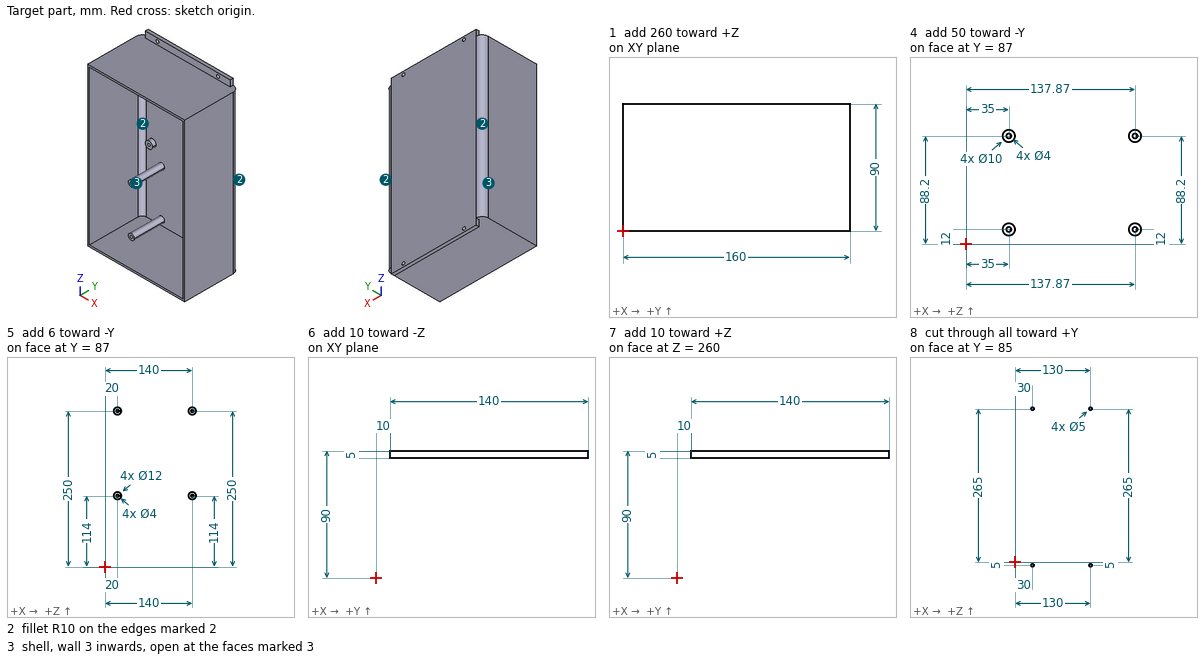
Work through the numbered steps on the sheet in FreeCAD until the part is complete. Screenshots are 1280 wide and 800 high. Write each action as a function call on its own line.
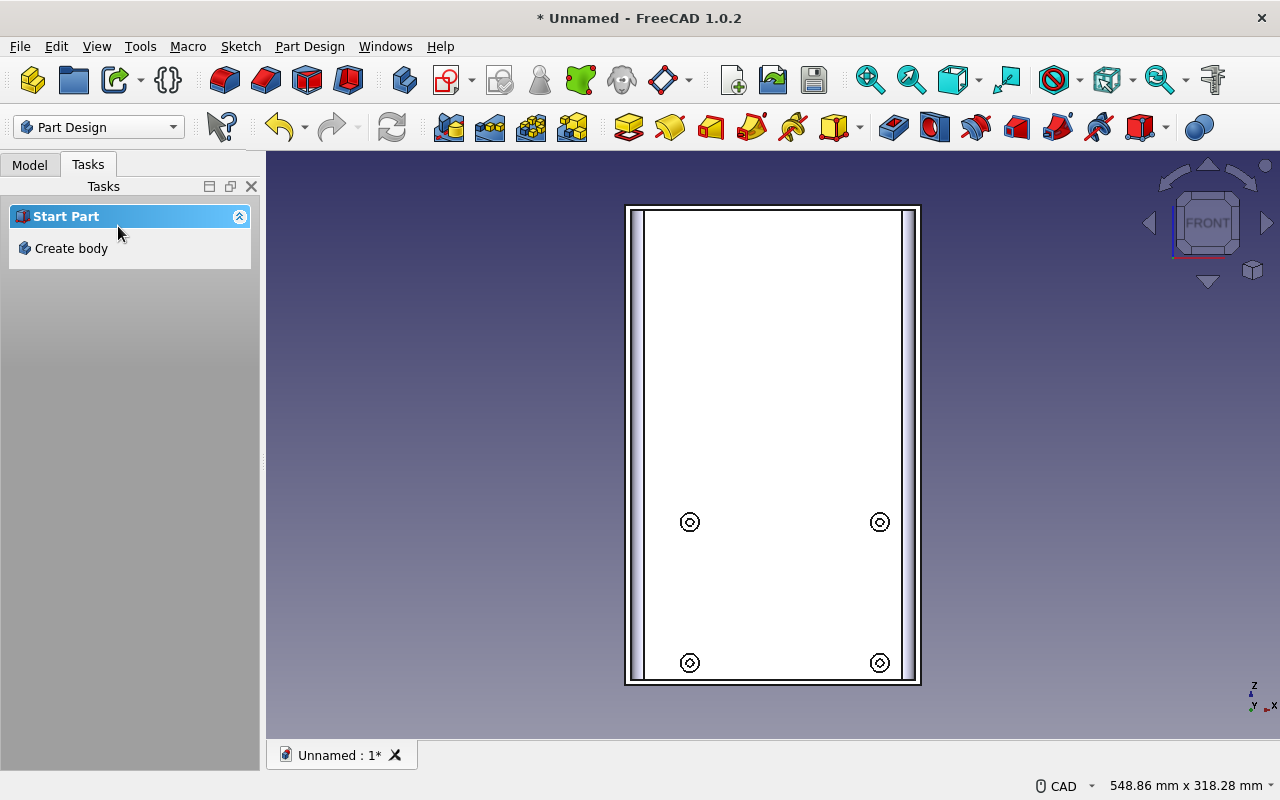
click(773, 377)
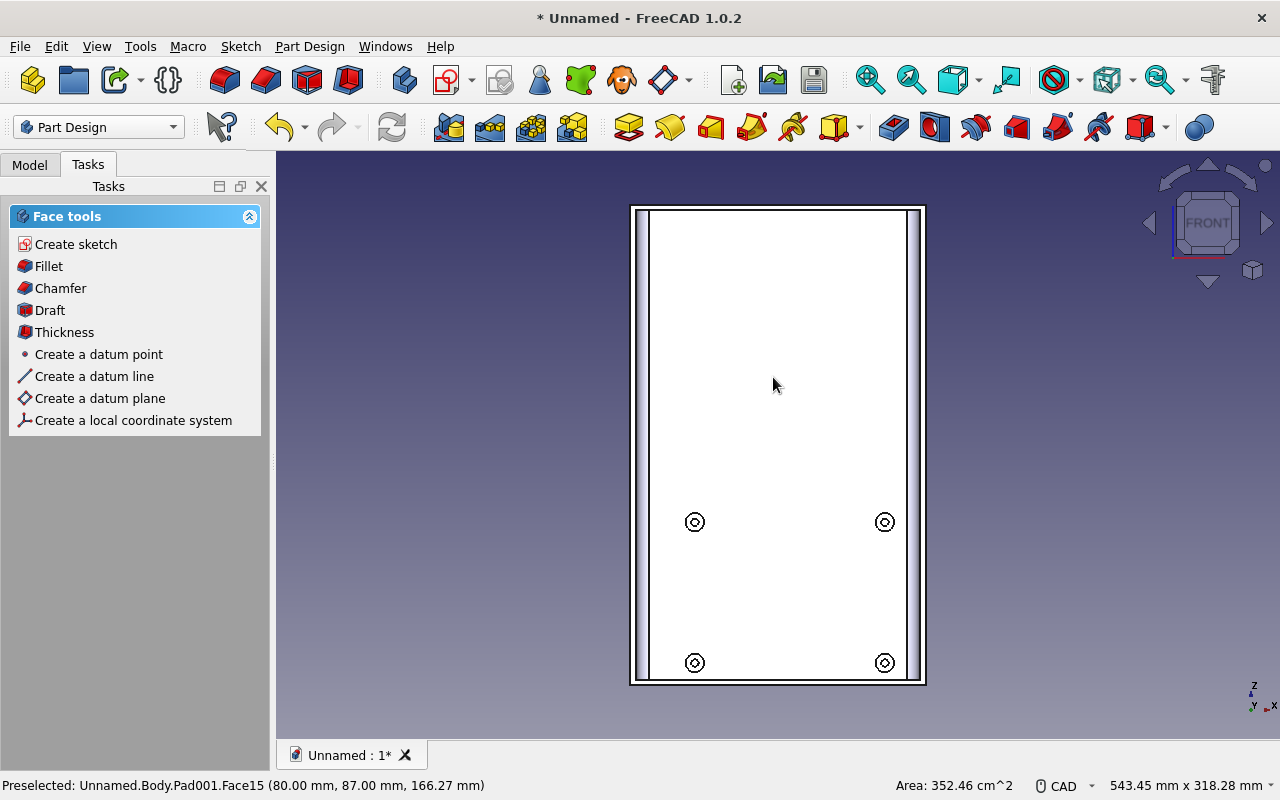
click(446, 80)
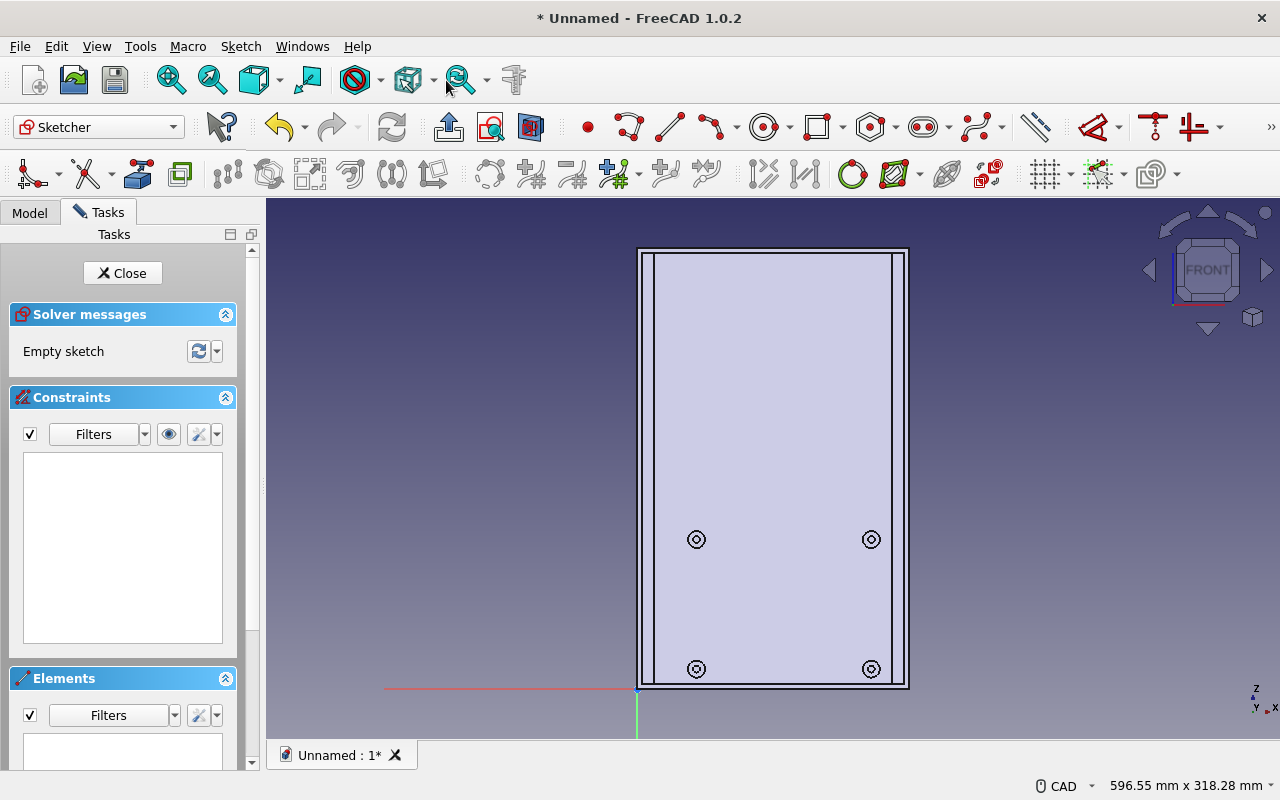
scroll(449, 453, down, 1)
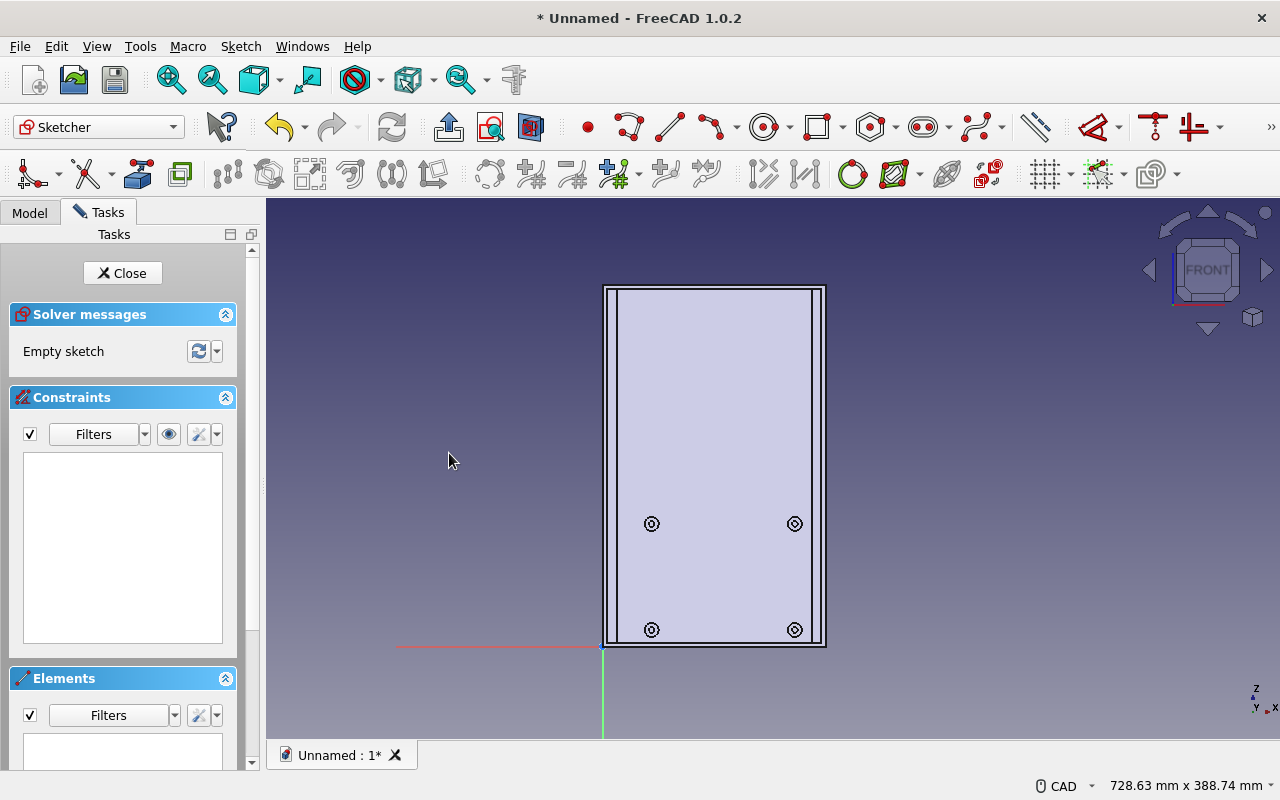
click(764, 128)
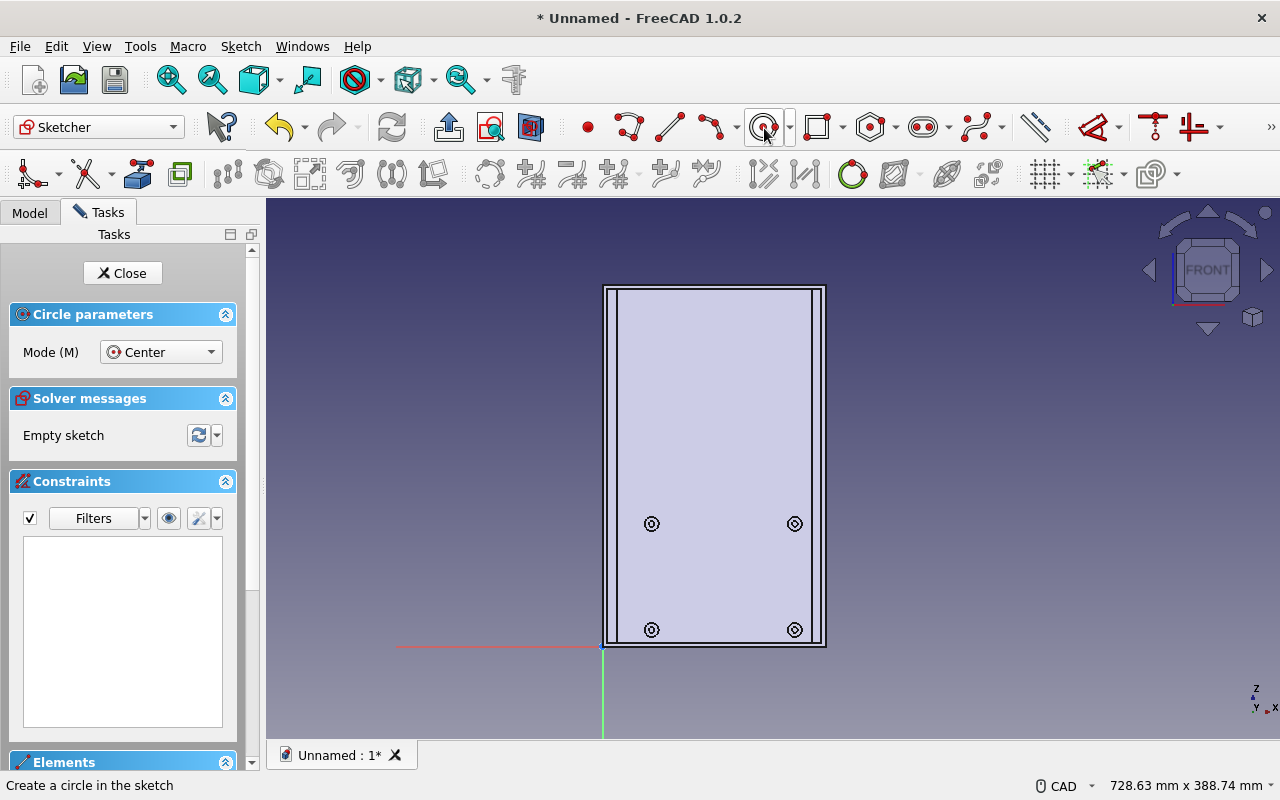
scroll(631, 488, up, 5)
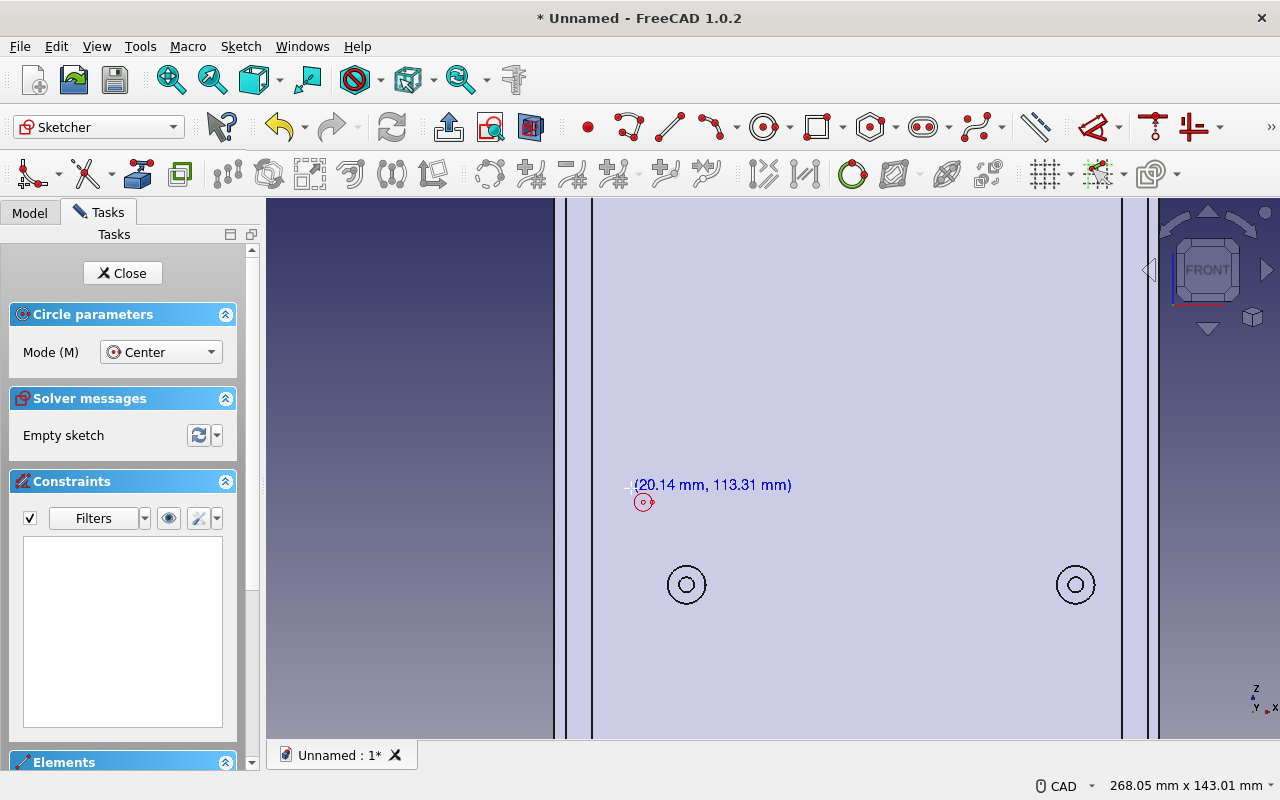
click(630, 487)
click(646, 471)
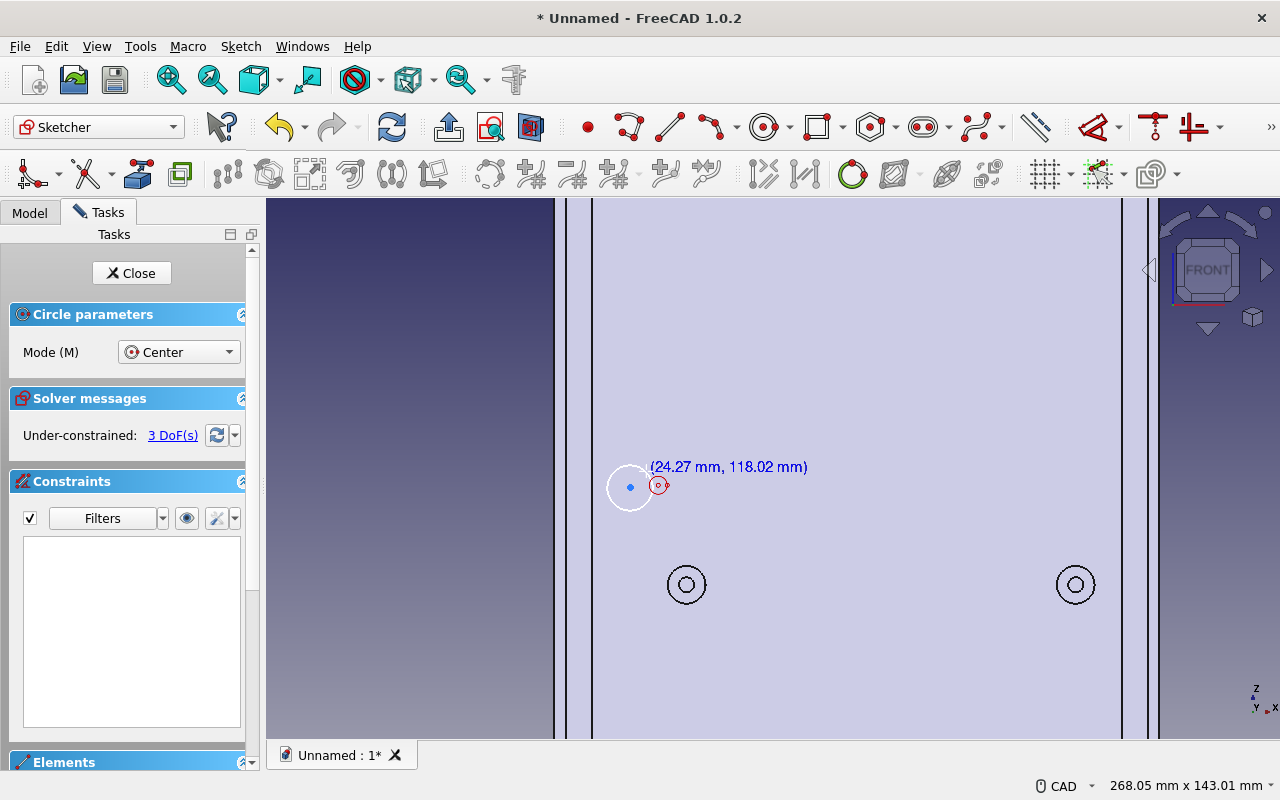
scroll(631, 488, down, 5)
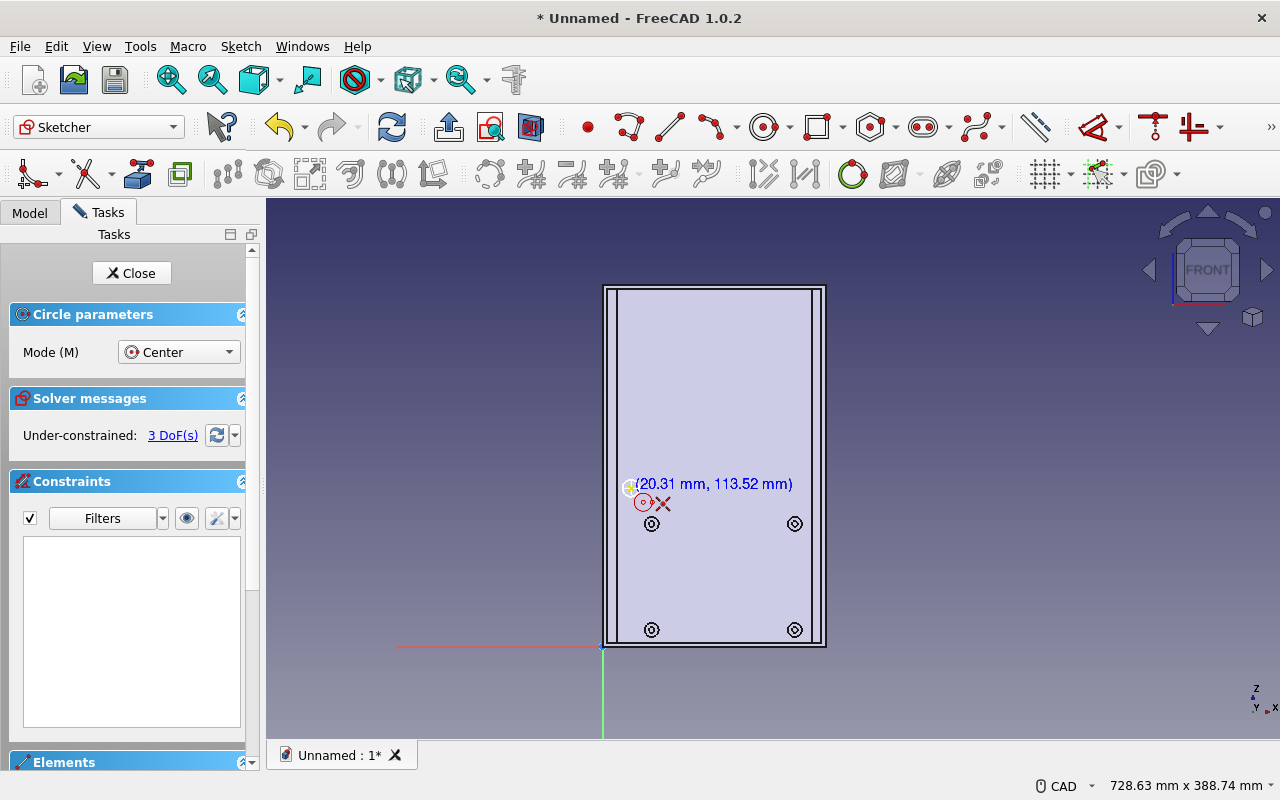
scroll(631, 299, up, 5)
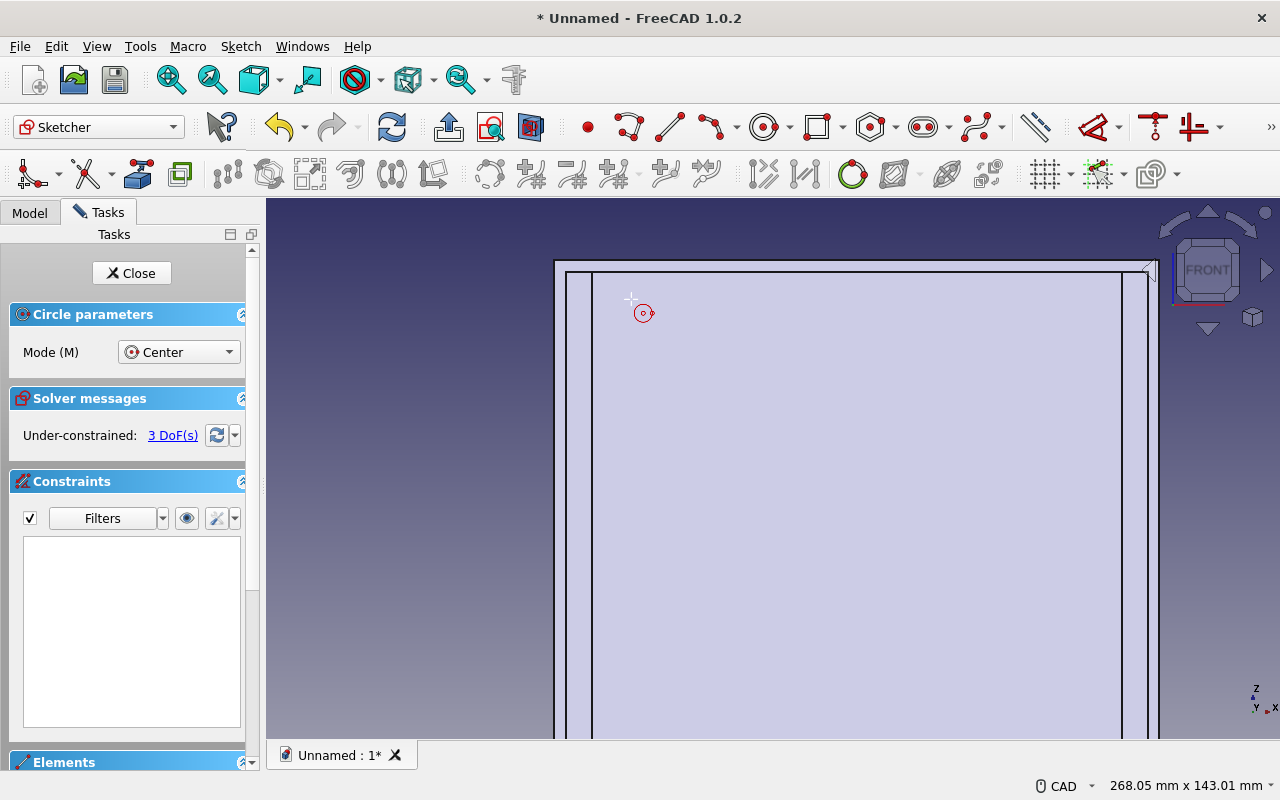
click(630, 298)
click(646, 282)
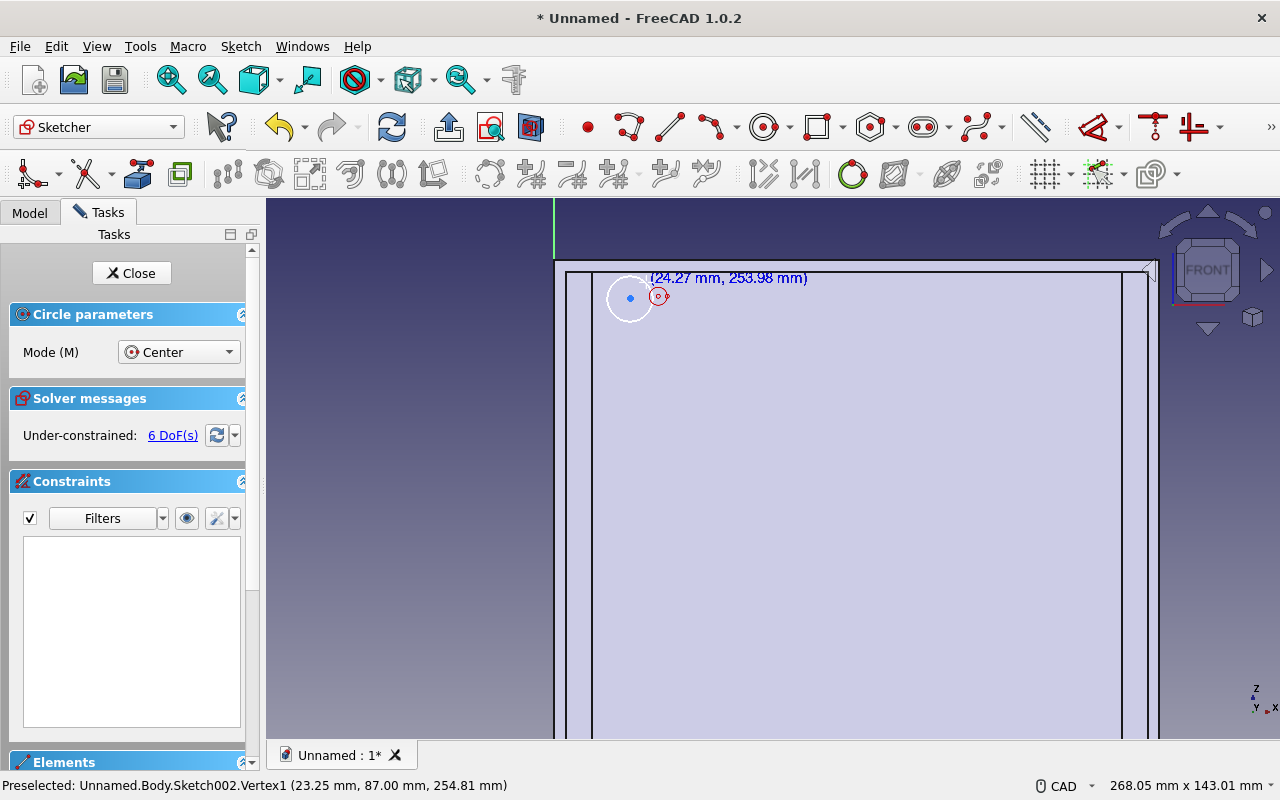
scroll(631, 299, down, 5)